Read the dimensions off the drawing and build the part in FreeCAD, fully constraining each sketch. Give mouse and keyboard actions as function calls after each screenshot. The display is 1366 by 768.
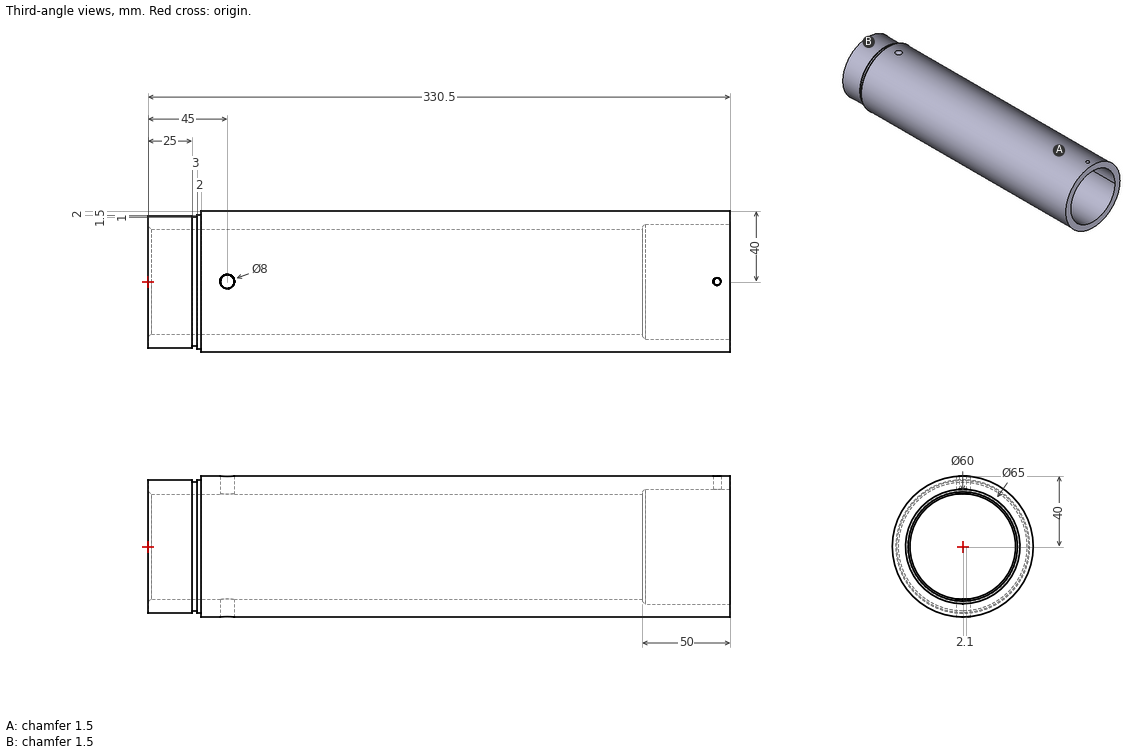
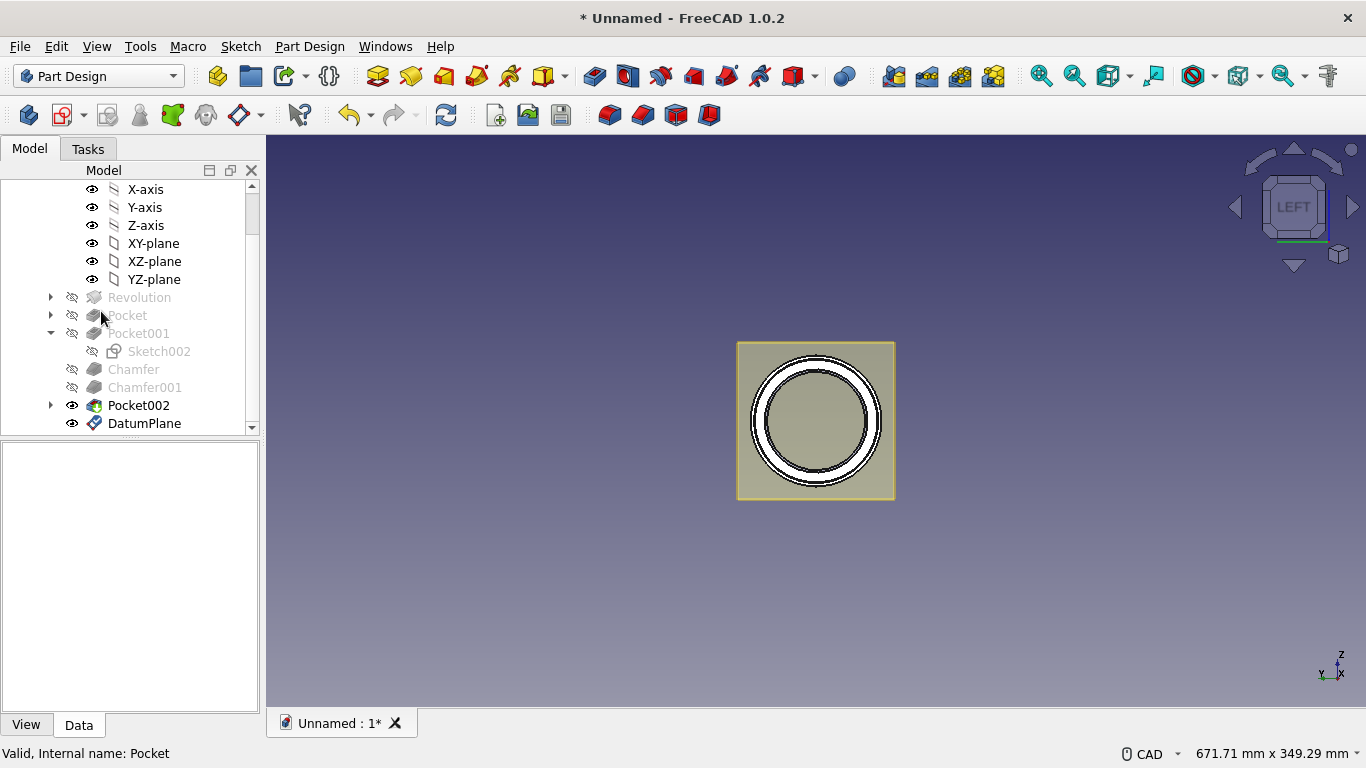
click(117, 423)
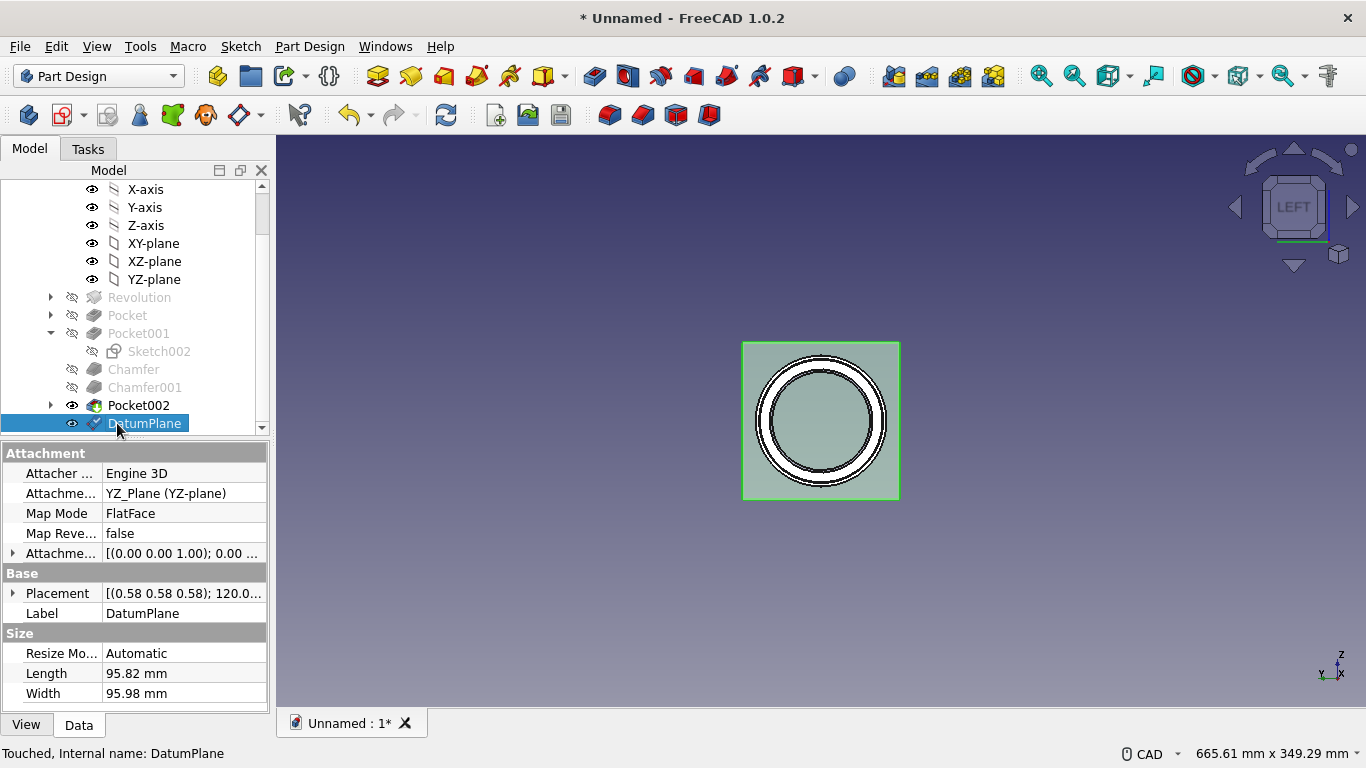
click(62, 116)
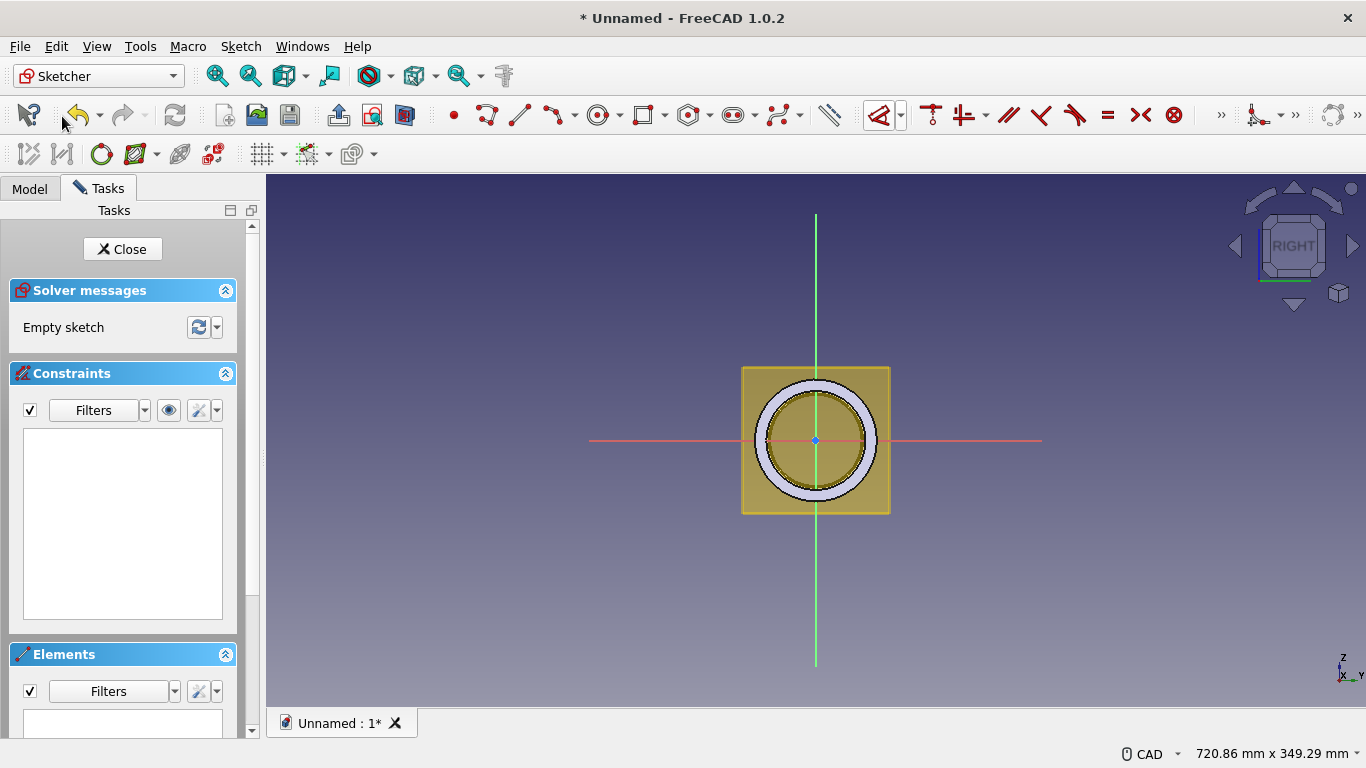
click(405, 116)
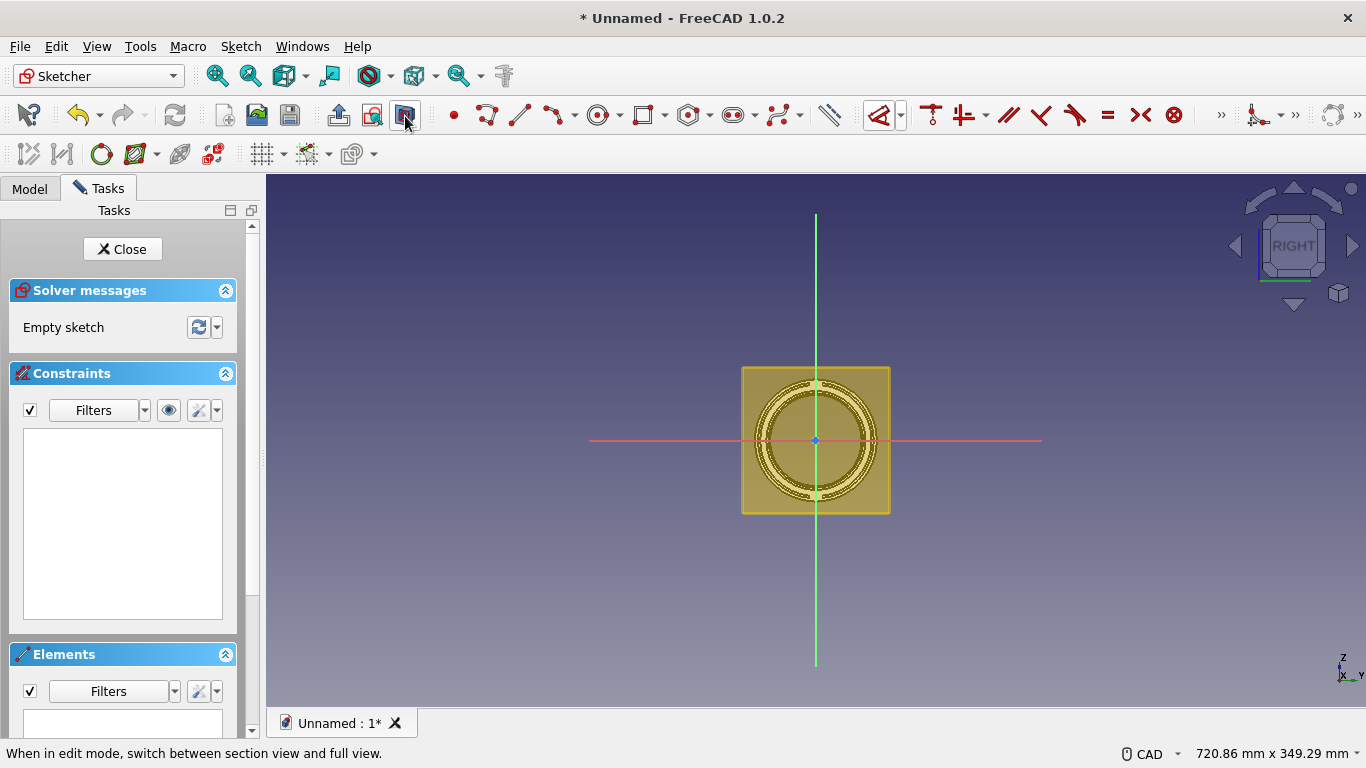
scroll(831, 404, up, 9)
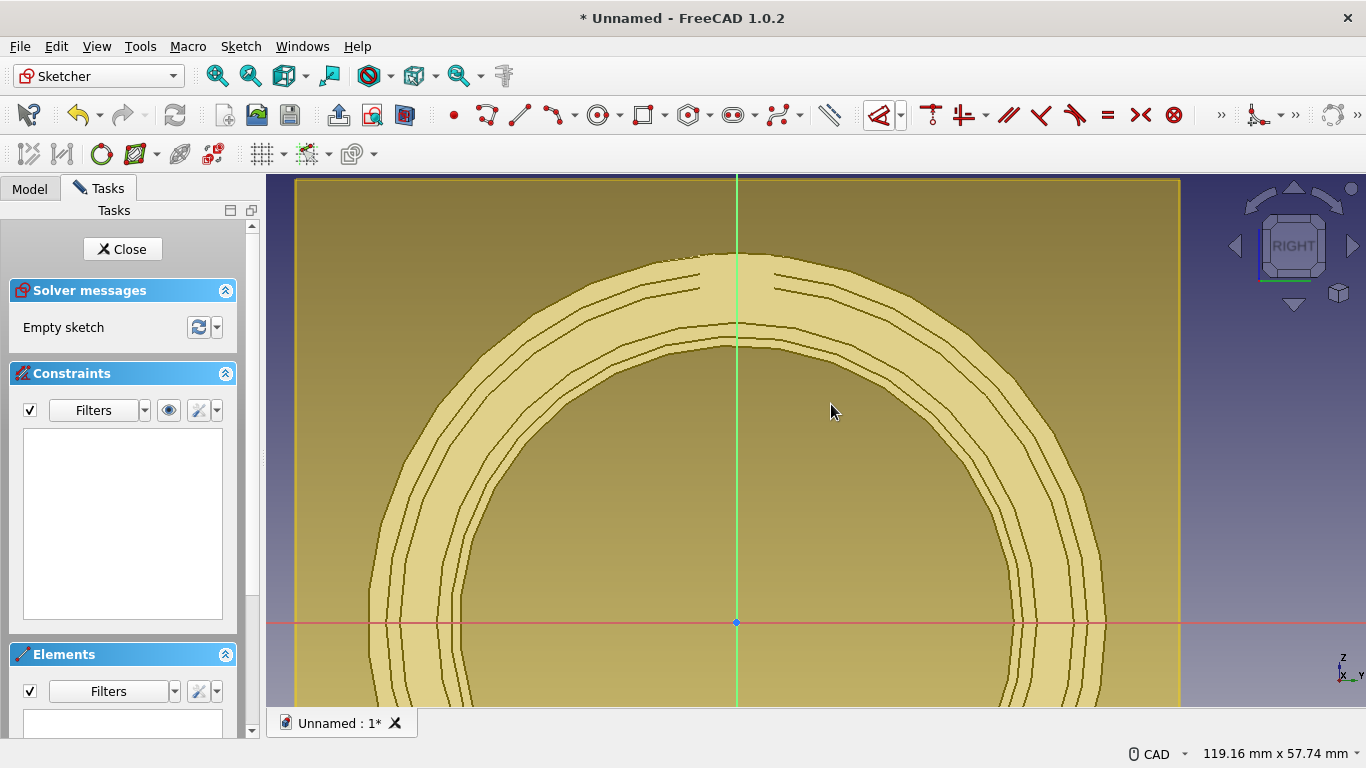
click(642, 116)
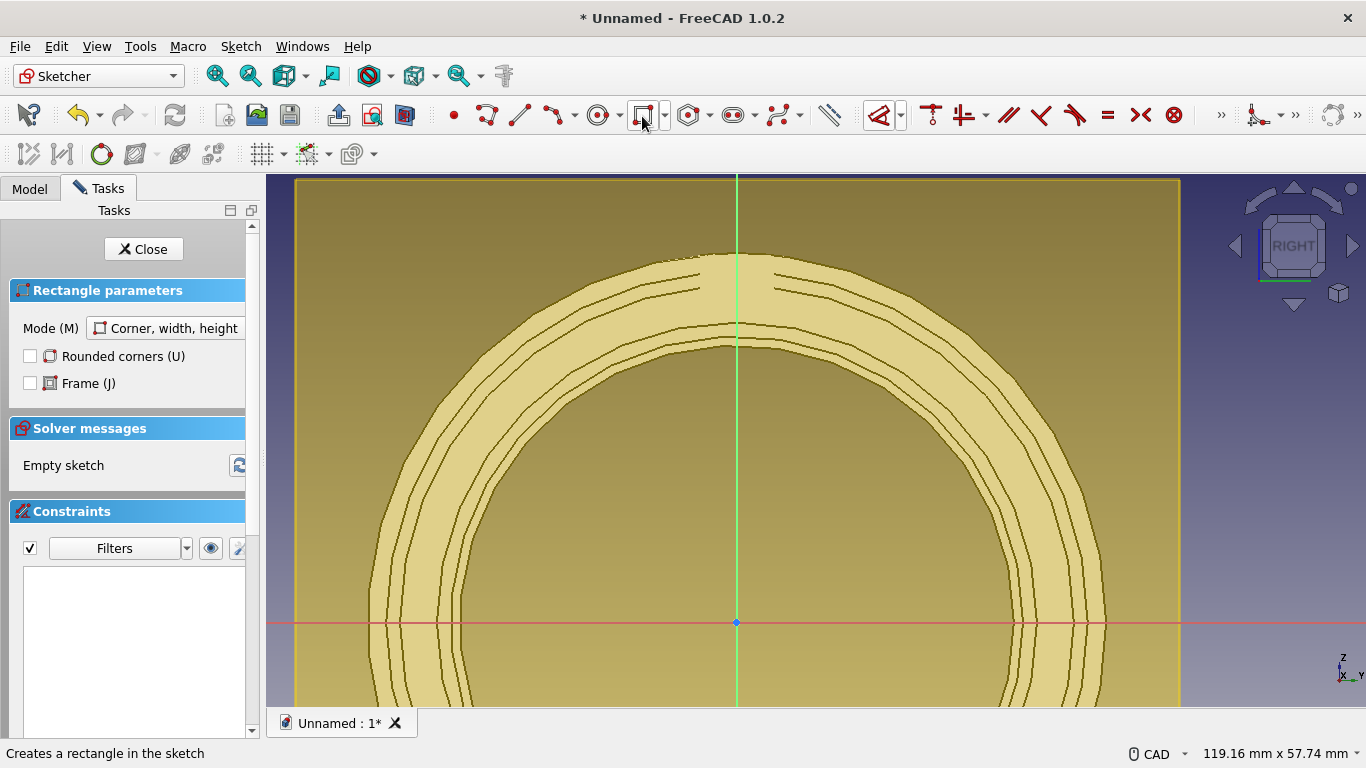
click(737, 623)
move(756, 253)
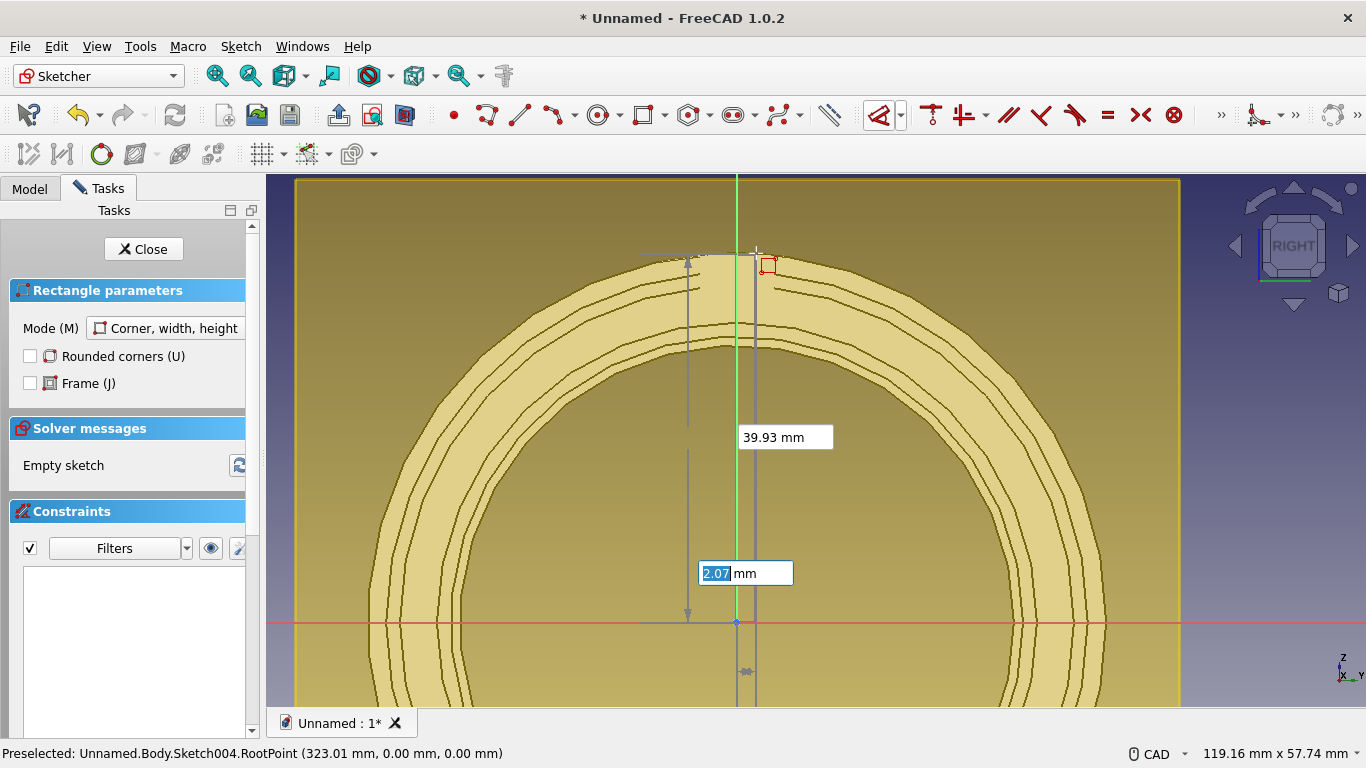
text(2.1)
key(Tab)
text(40)
key(Return)
key(Escape)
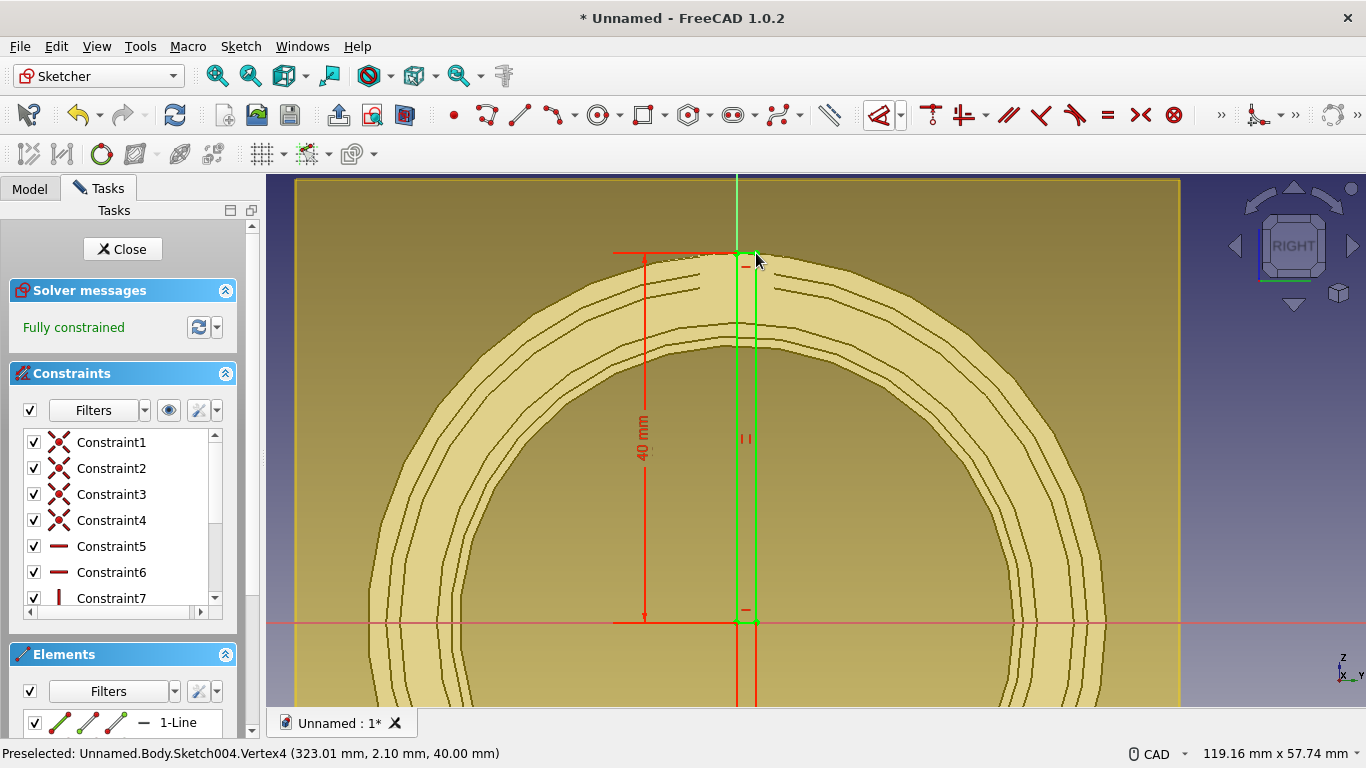
click(123, 249)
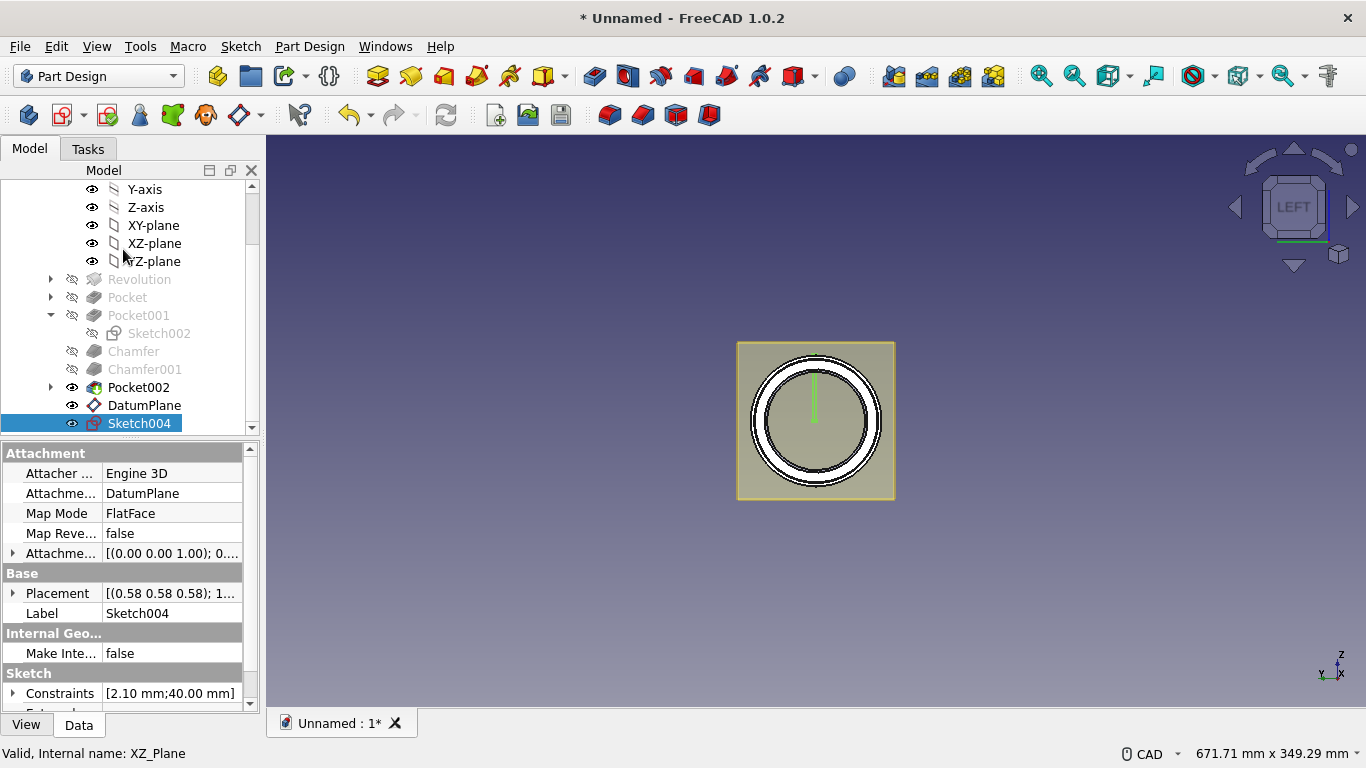
click(661, 76)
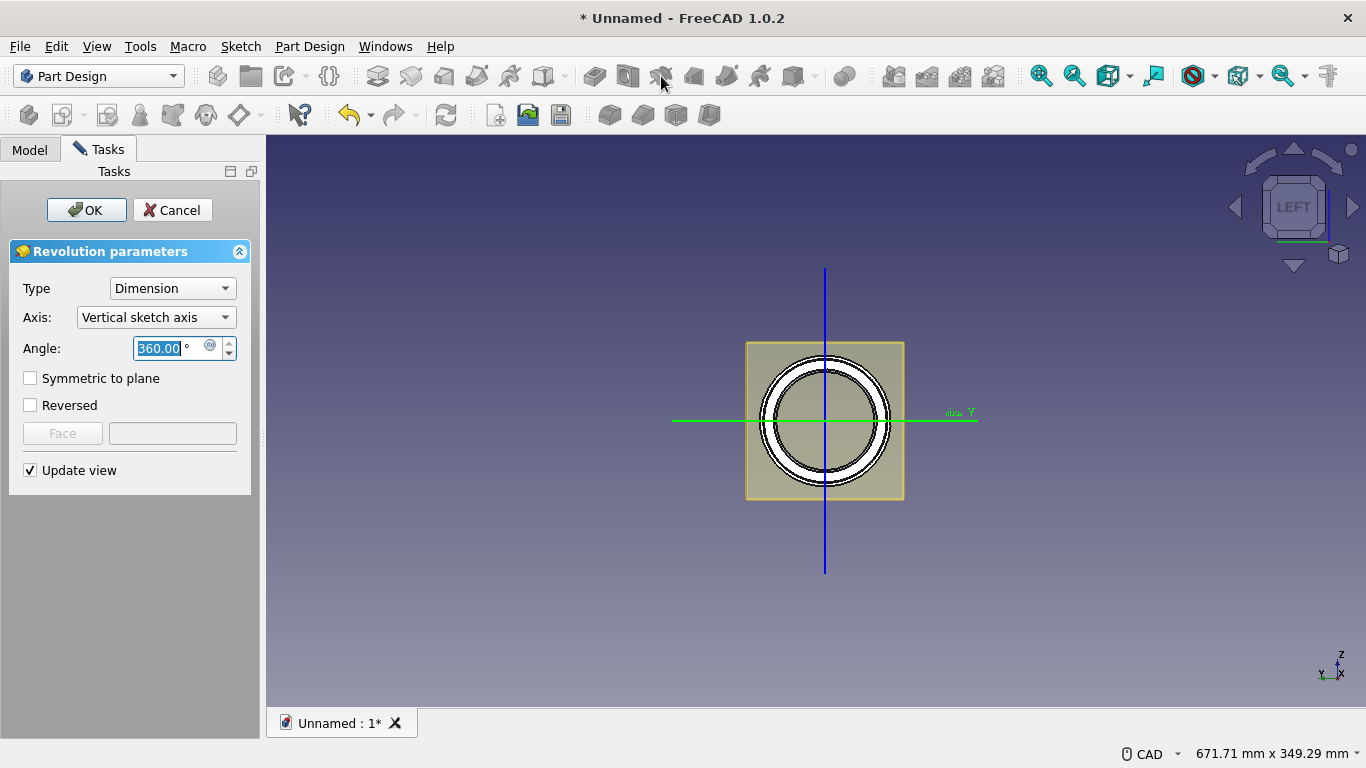
click(87, 210)